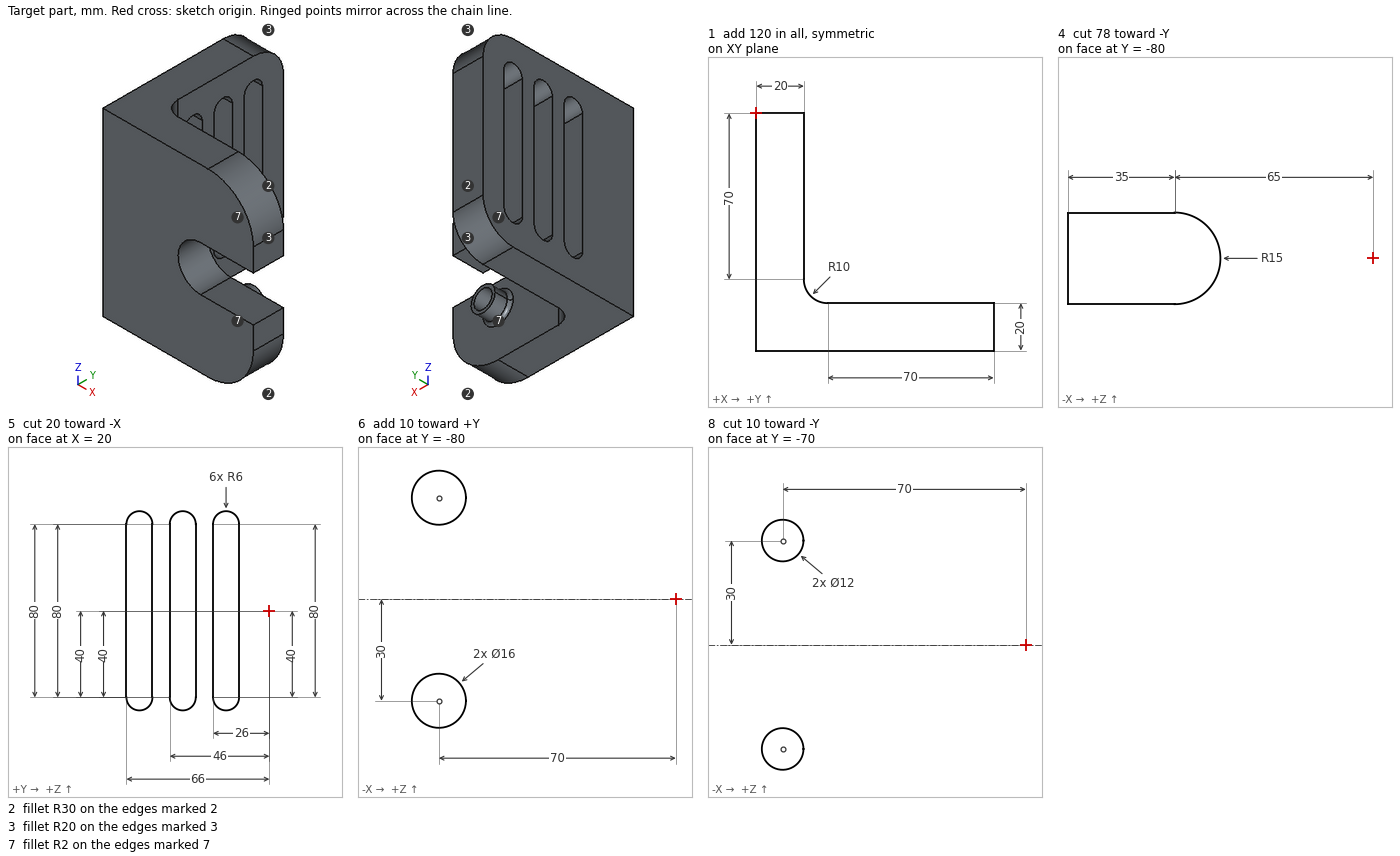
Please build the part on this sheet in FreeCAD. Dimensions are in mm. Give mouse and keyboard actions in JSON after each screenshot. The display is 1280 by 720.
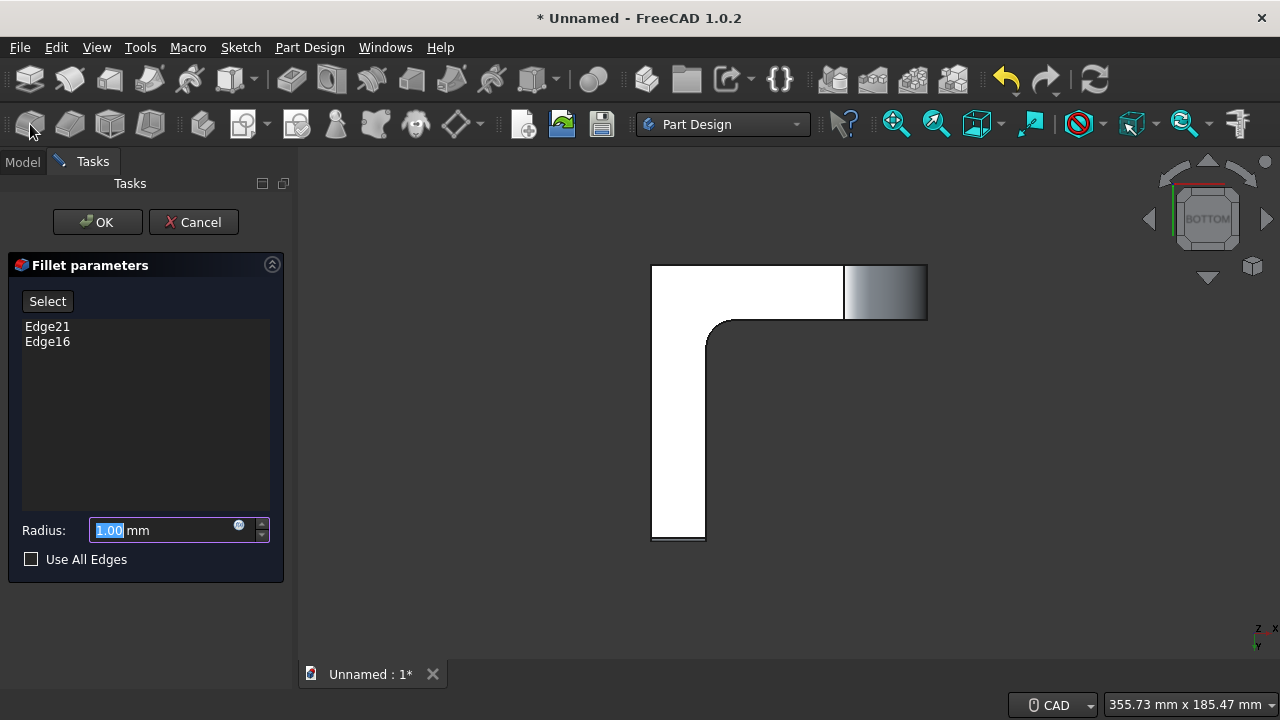
{"action": "type", "text": "20"}
{"action": "key", "text": "Tab"}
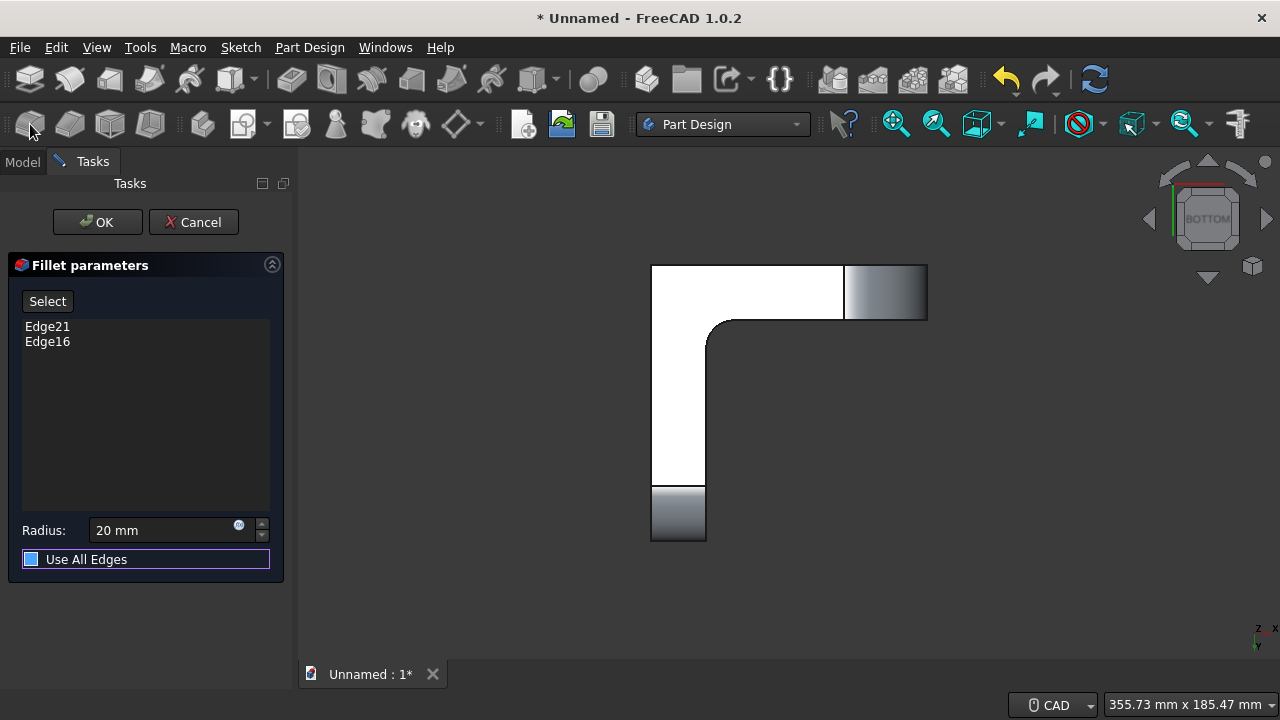
{"action": "left_click", "coordinate": [98, 222]}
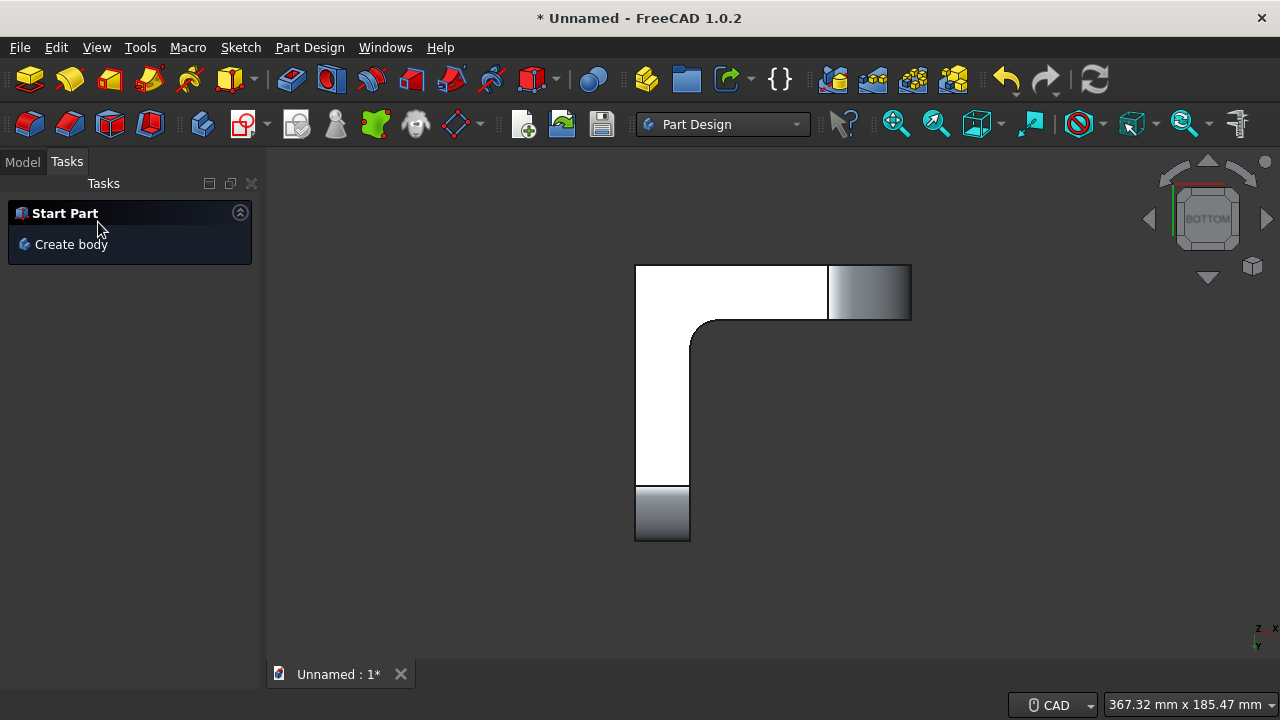
{"action": "key", "text": "4"}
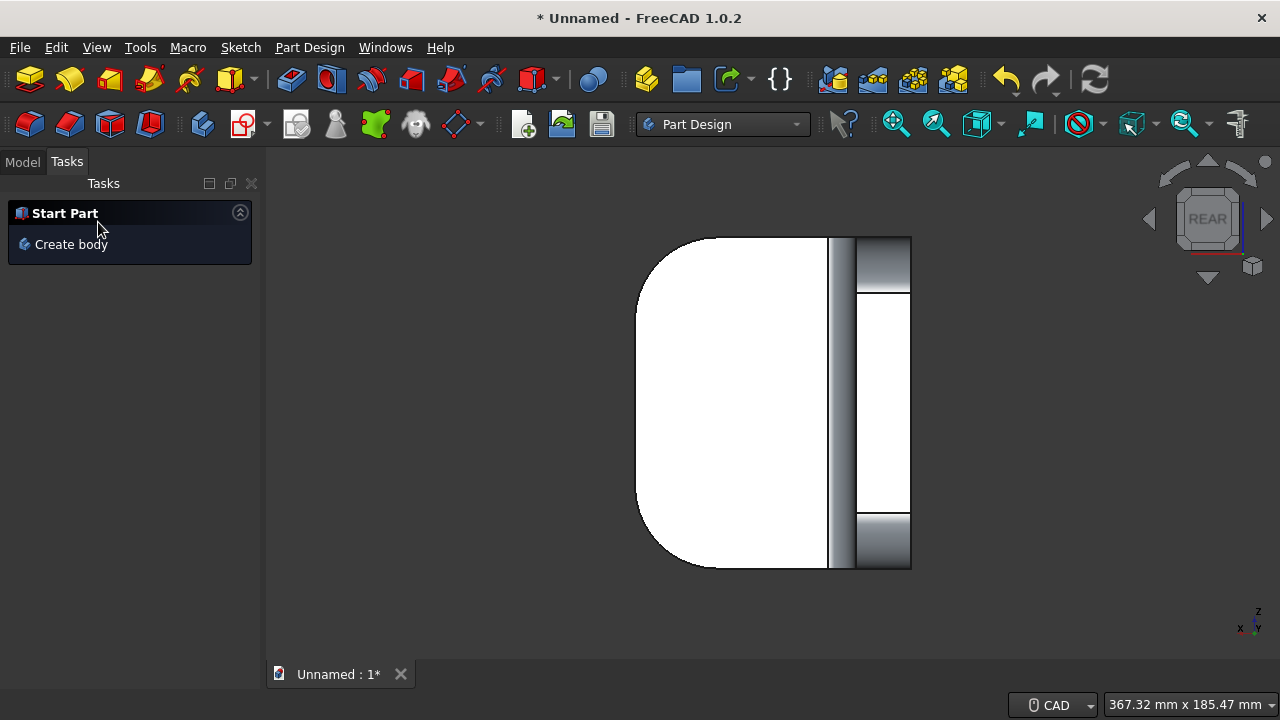
{"action": "left_click", "coordinate": [732, 355]}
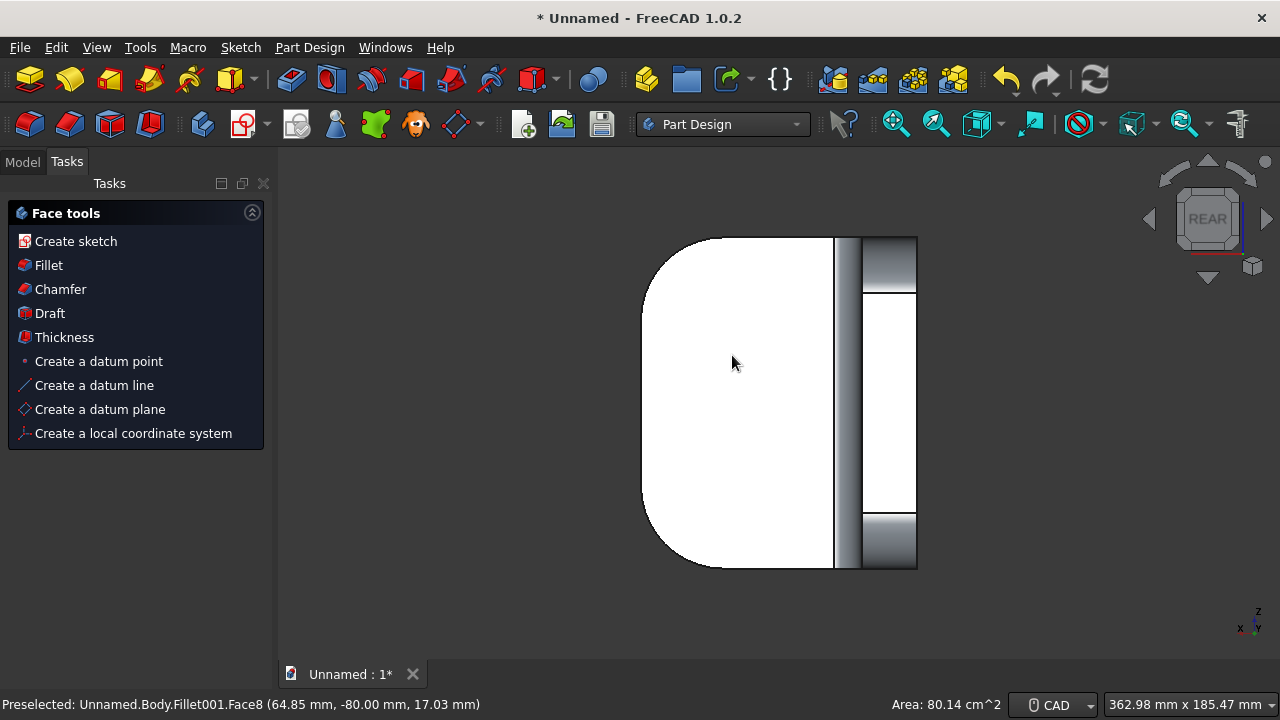
{"action": "left_click", "coordinate": [244, 124]}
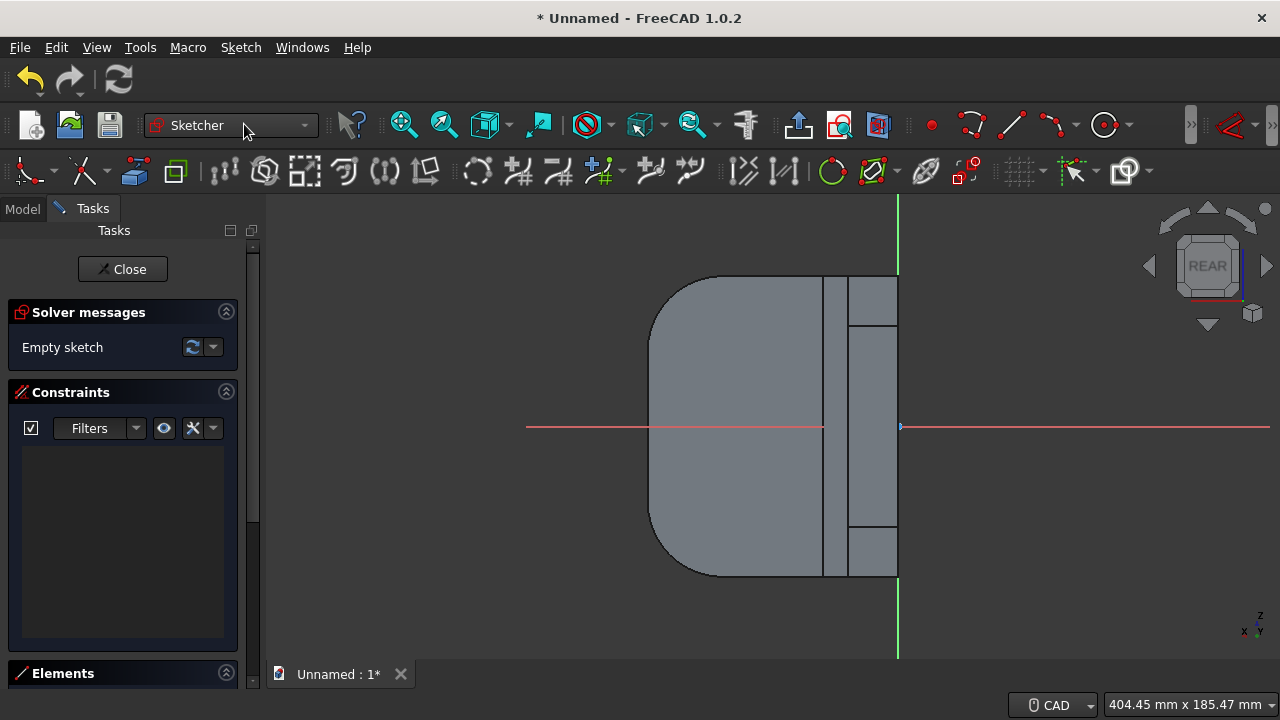
{"action": "key", "text": "q s"}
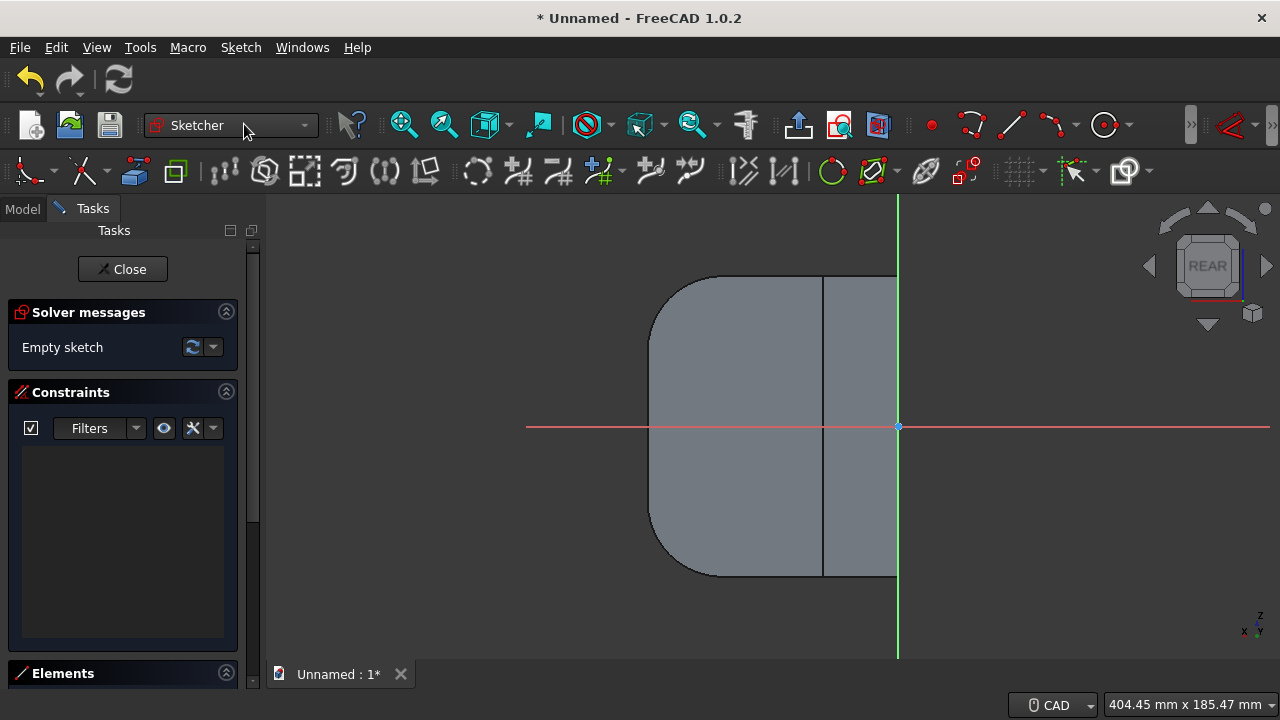
{"action": "scroll", "coordinate": [829, 426], "scroll_direction": "up", "scroll_amount": 4}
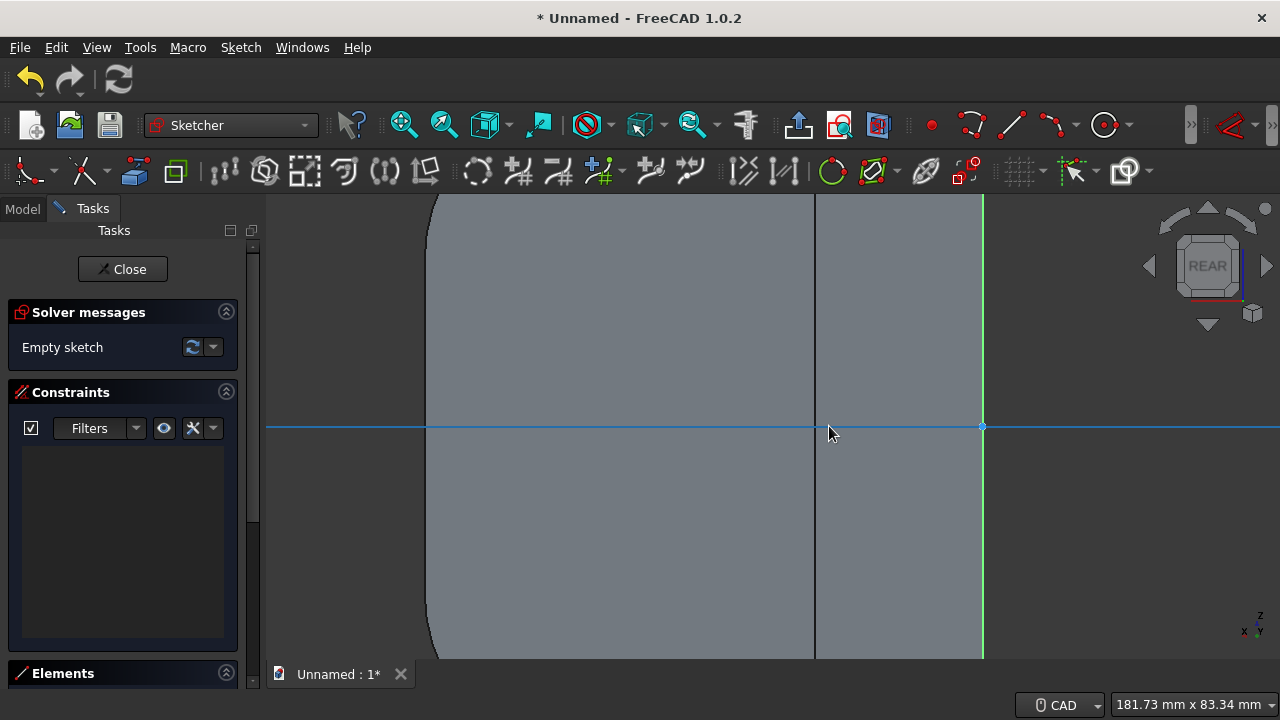
{"action": "key", "text": "g m"}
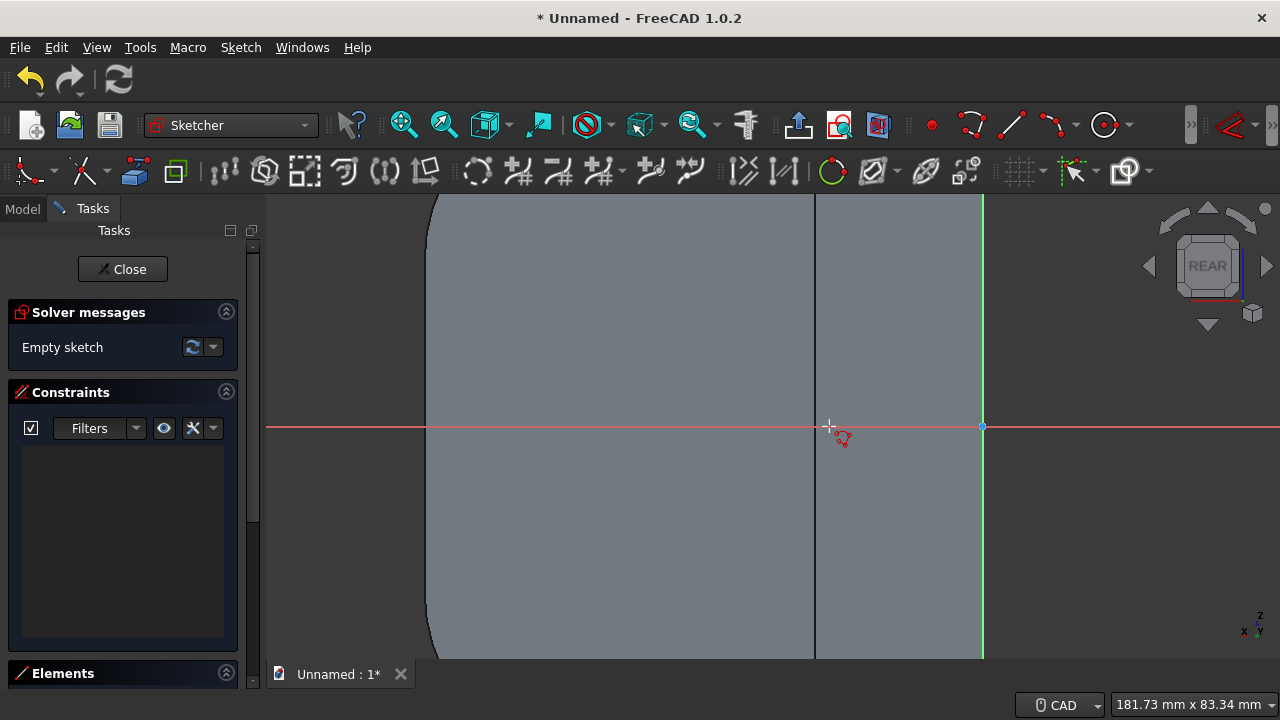
{"action": "left_click", "coordinate": [620, 343]}
{"action": "left_click", "coordinate": [425, 343]}
{"action": "left_click", "coordinate": [425, 510]}
{"action": "left_click", "coordinate": [620, 510]}
{"action": "right_click", "coordinate": [620, 510]}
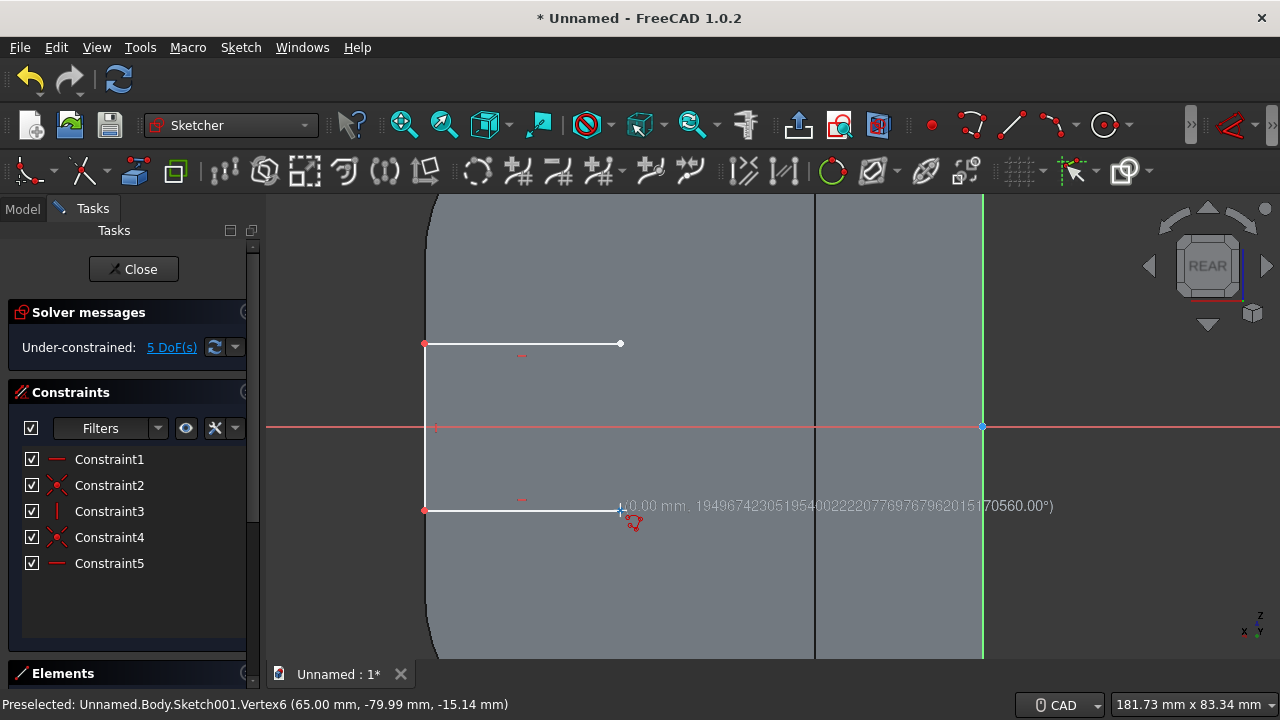
{"action": "left_click", "coordinate": [1052, 126]}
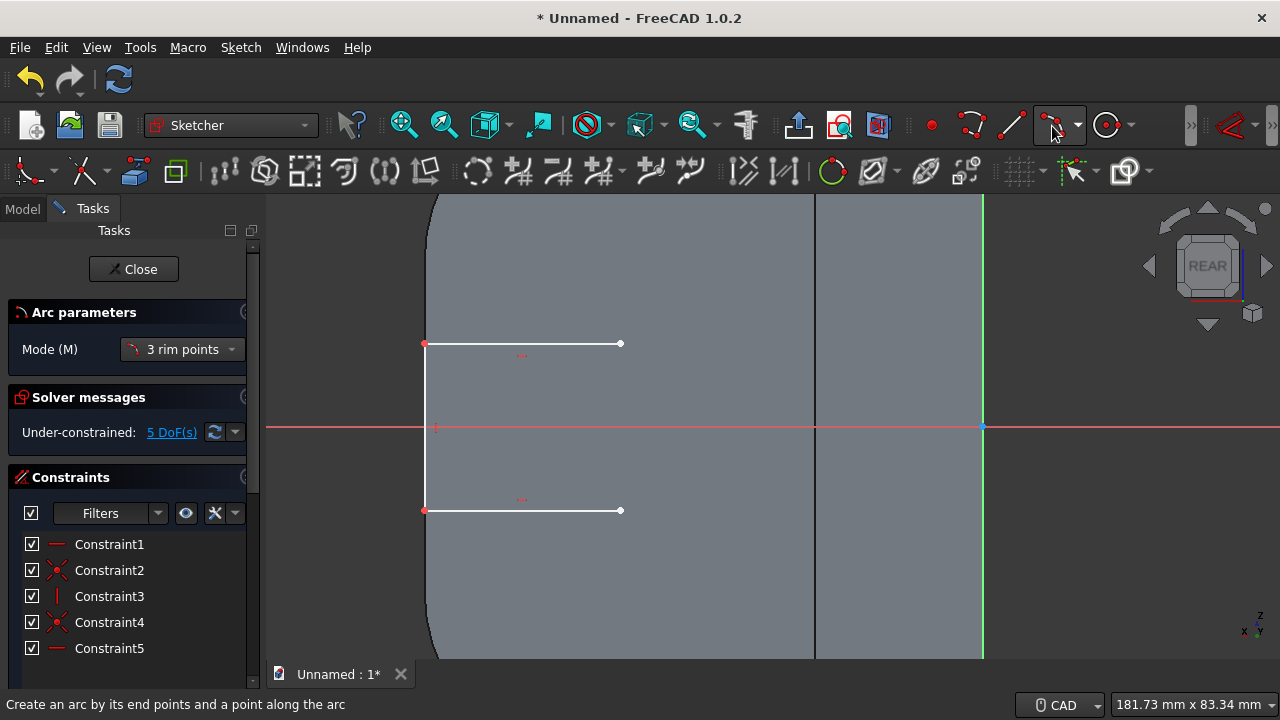
{"action": "left_click", "coordinate": [620, 511]}
{"action": "left_click", "coordinate": [620, 344]}
{"action": "left_click", "coordinate": [700, 452]}
{"action": "key", "text": "Escape"}